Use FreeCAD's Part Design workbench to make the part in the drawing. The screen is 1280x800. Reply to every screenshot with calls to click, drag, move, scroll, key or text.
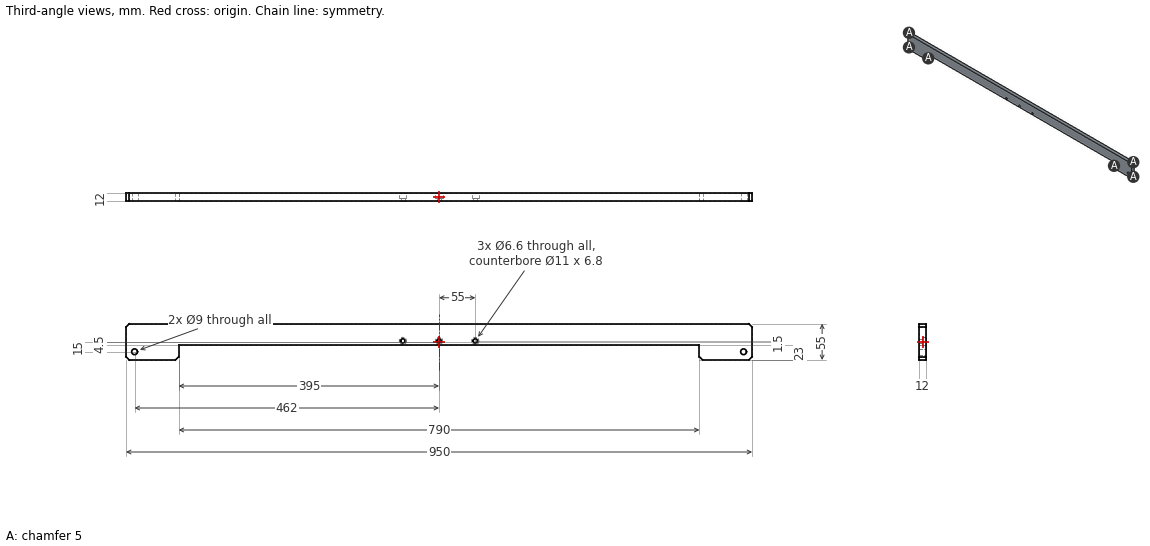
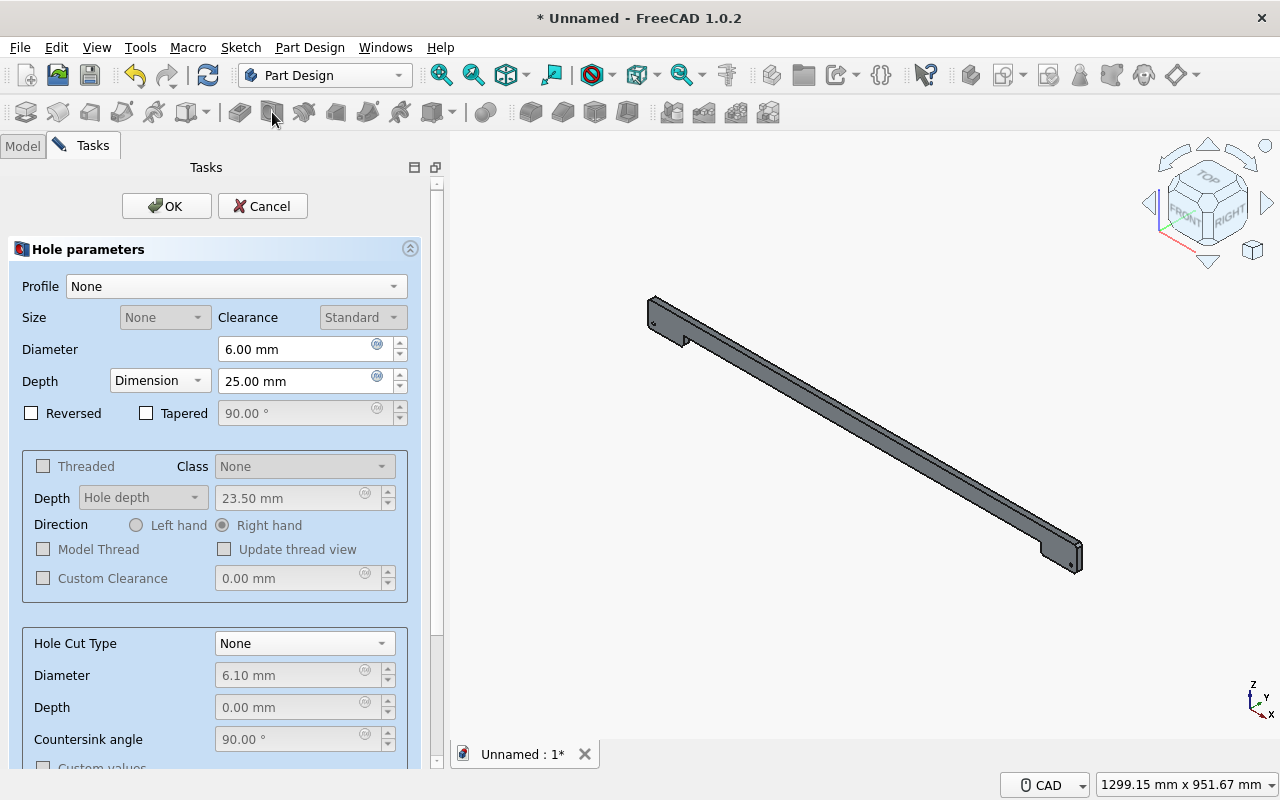
triple_click(305, 349)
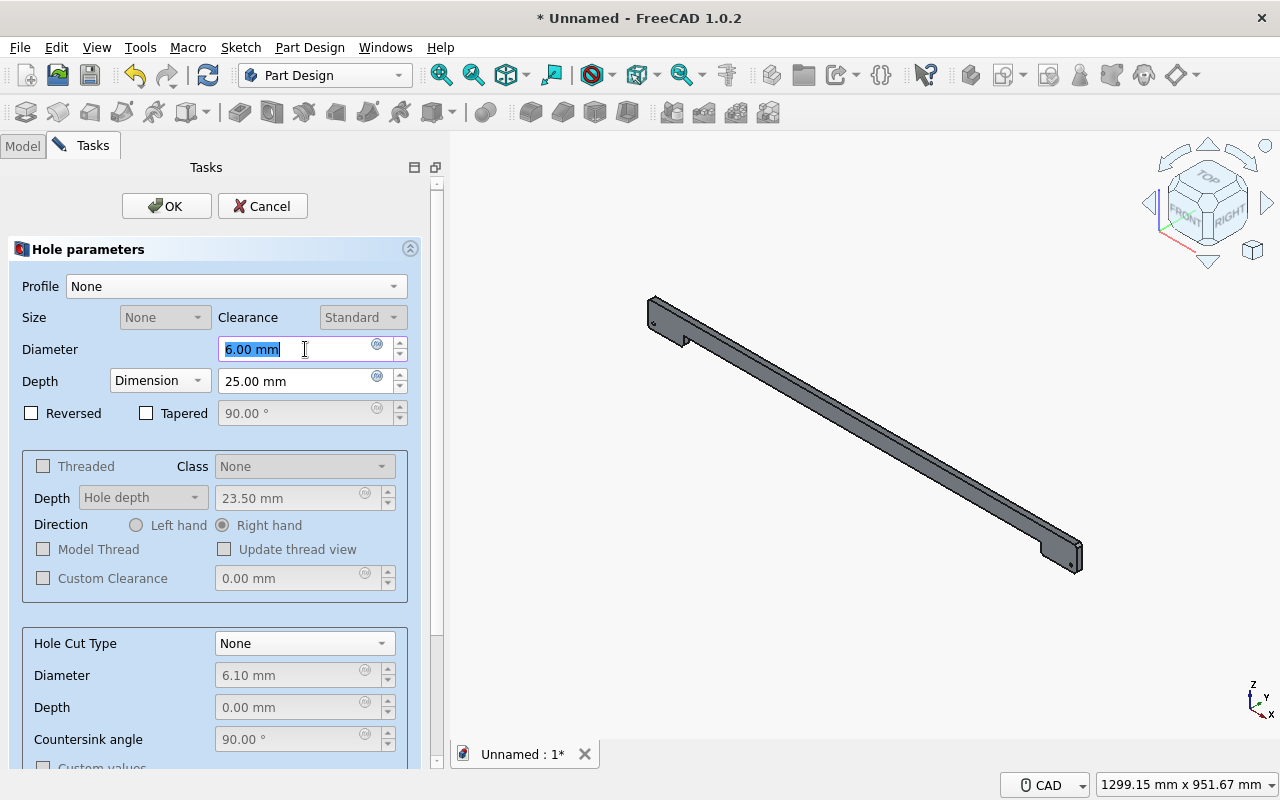
text(9)
key(Tab)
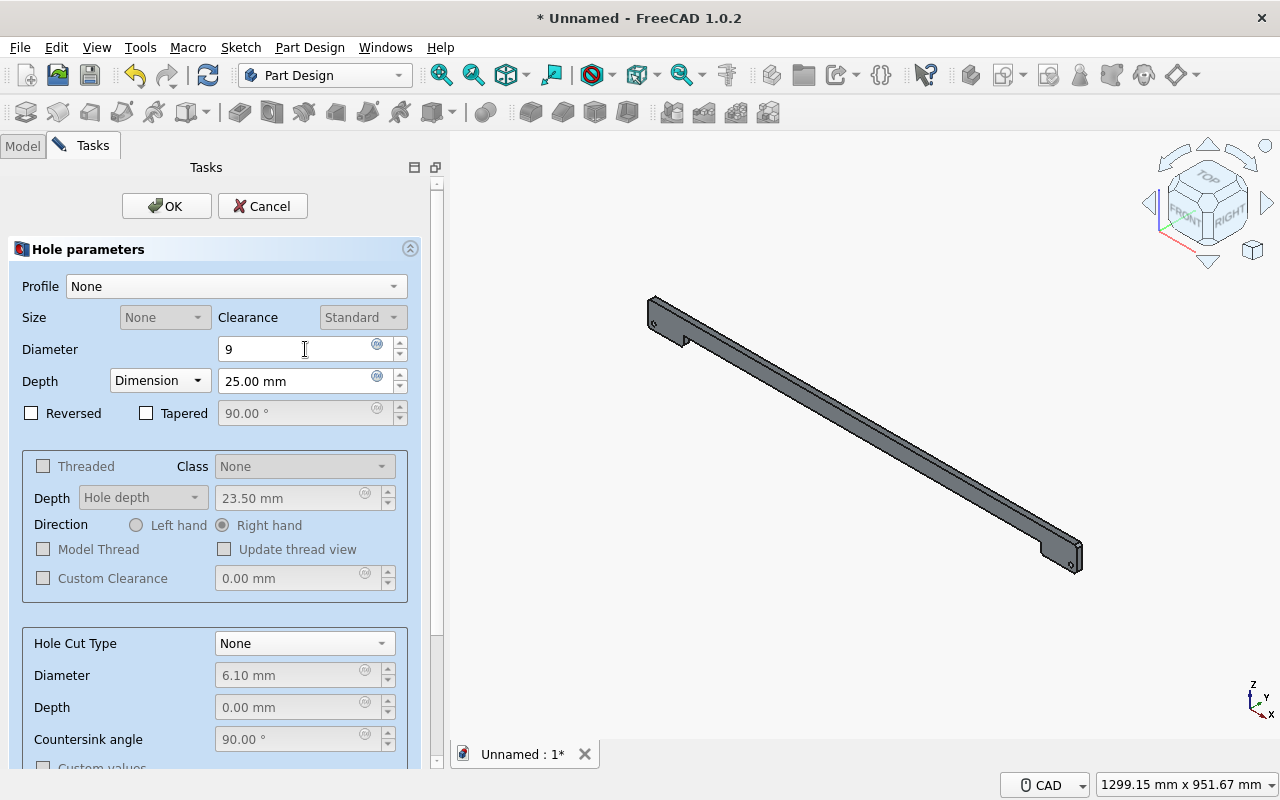
click(161, 380)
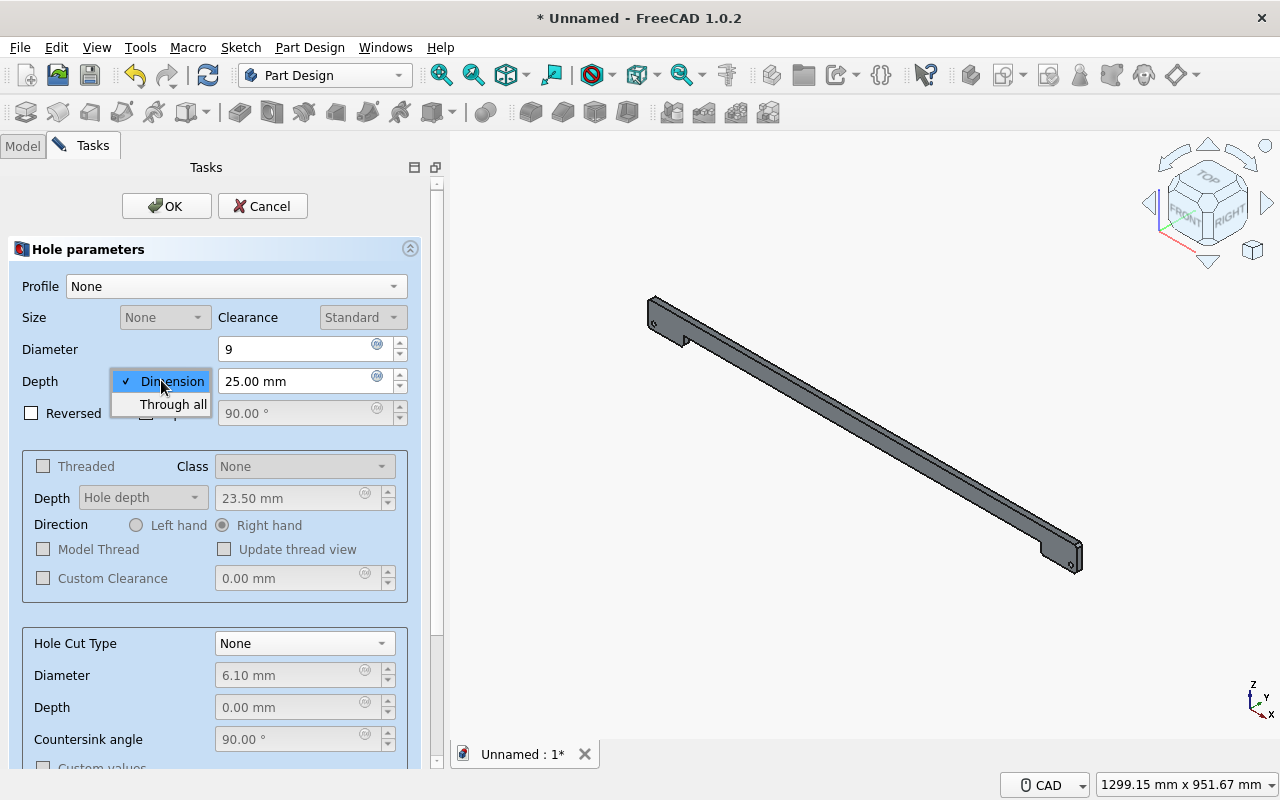
click(160, 404)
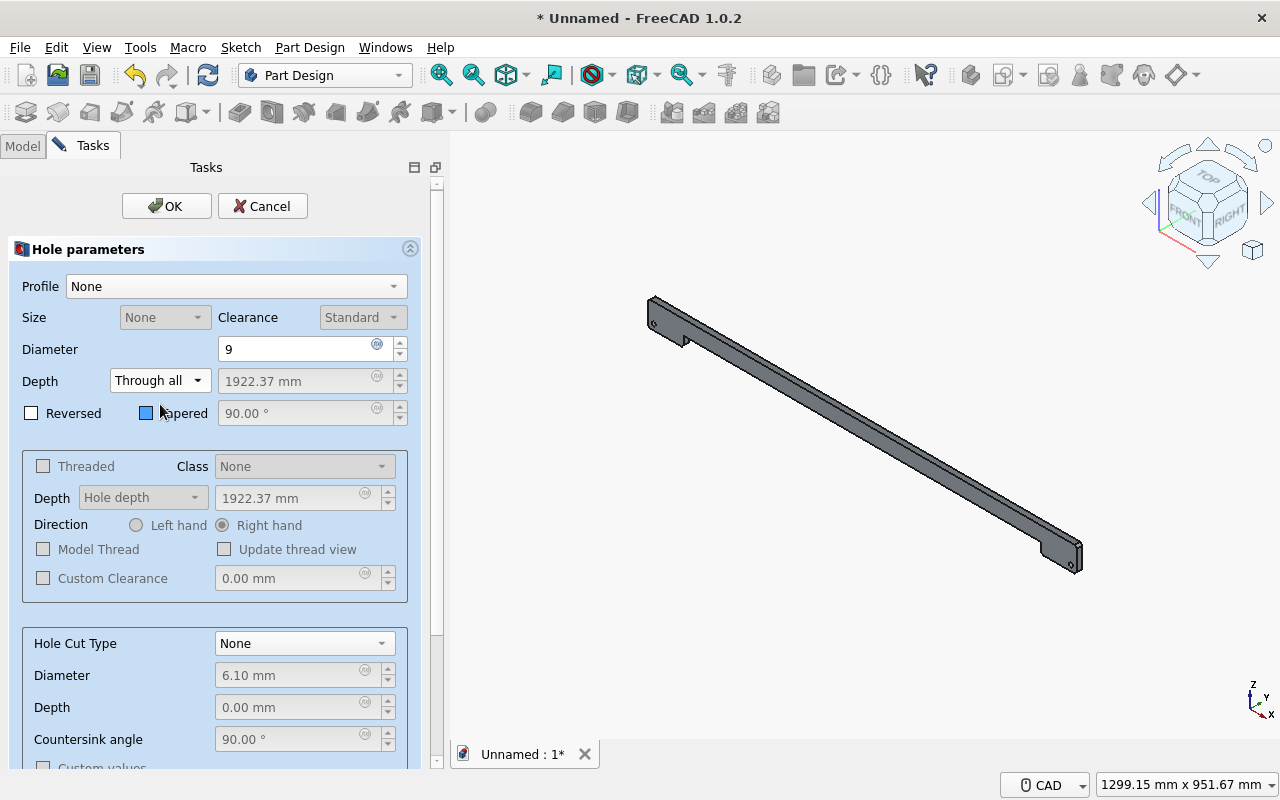
click(167, 206)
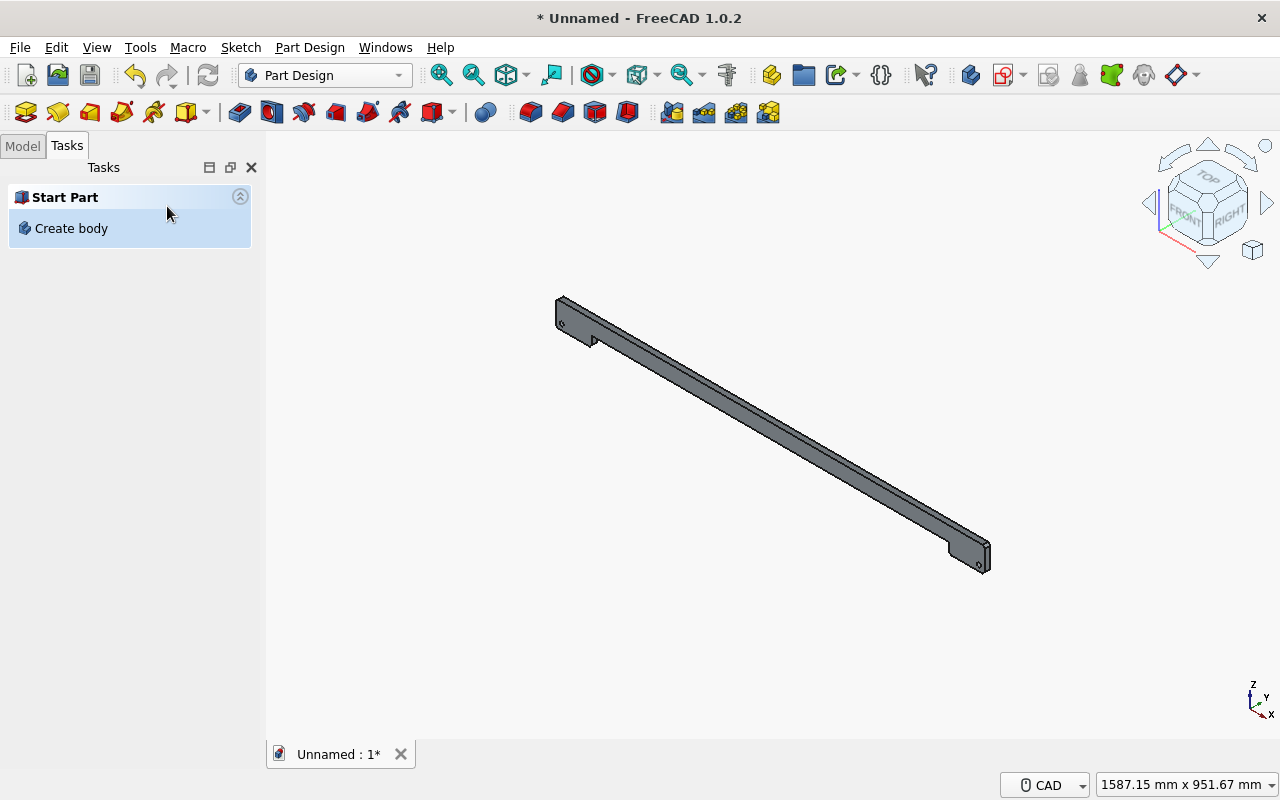
key(4)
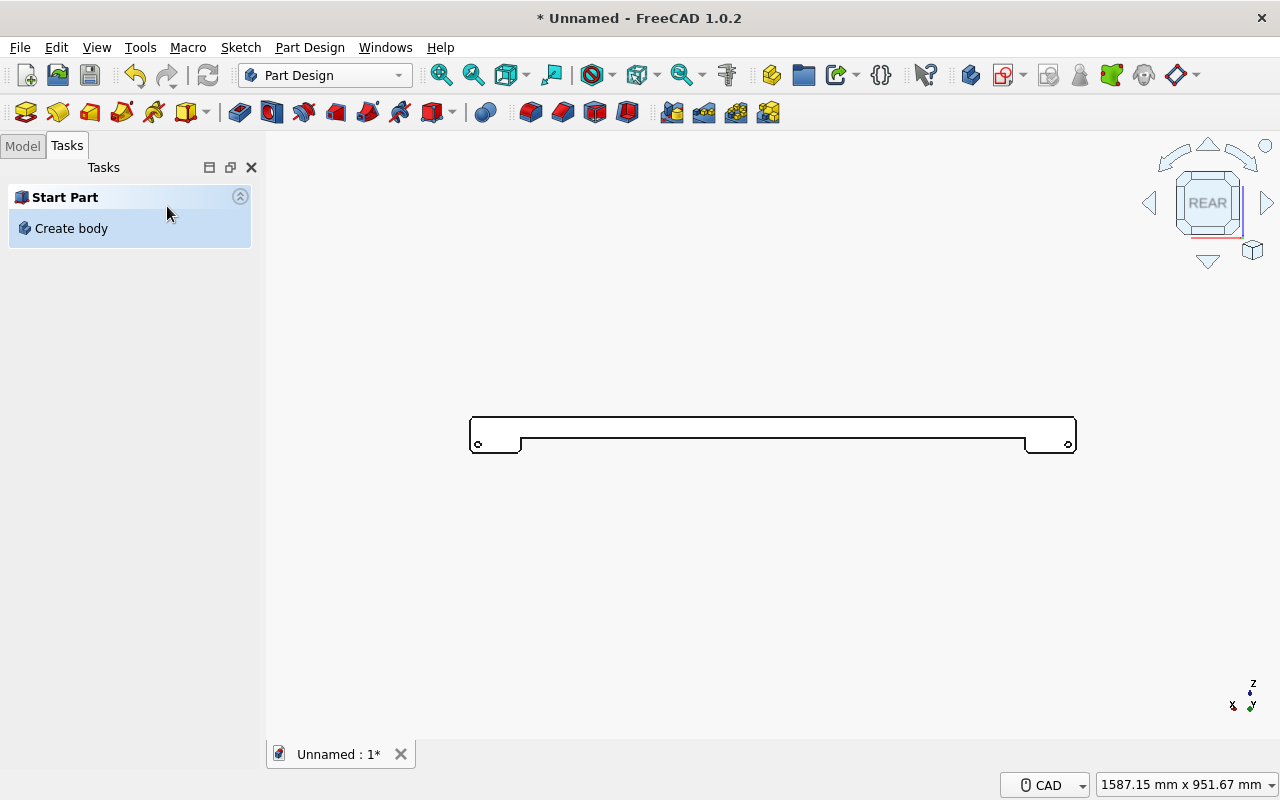
click(513, 429)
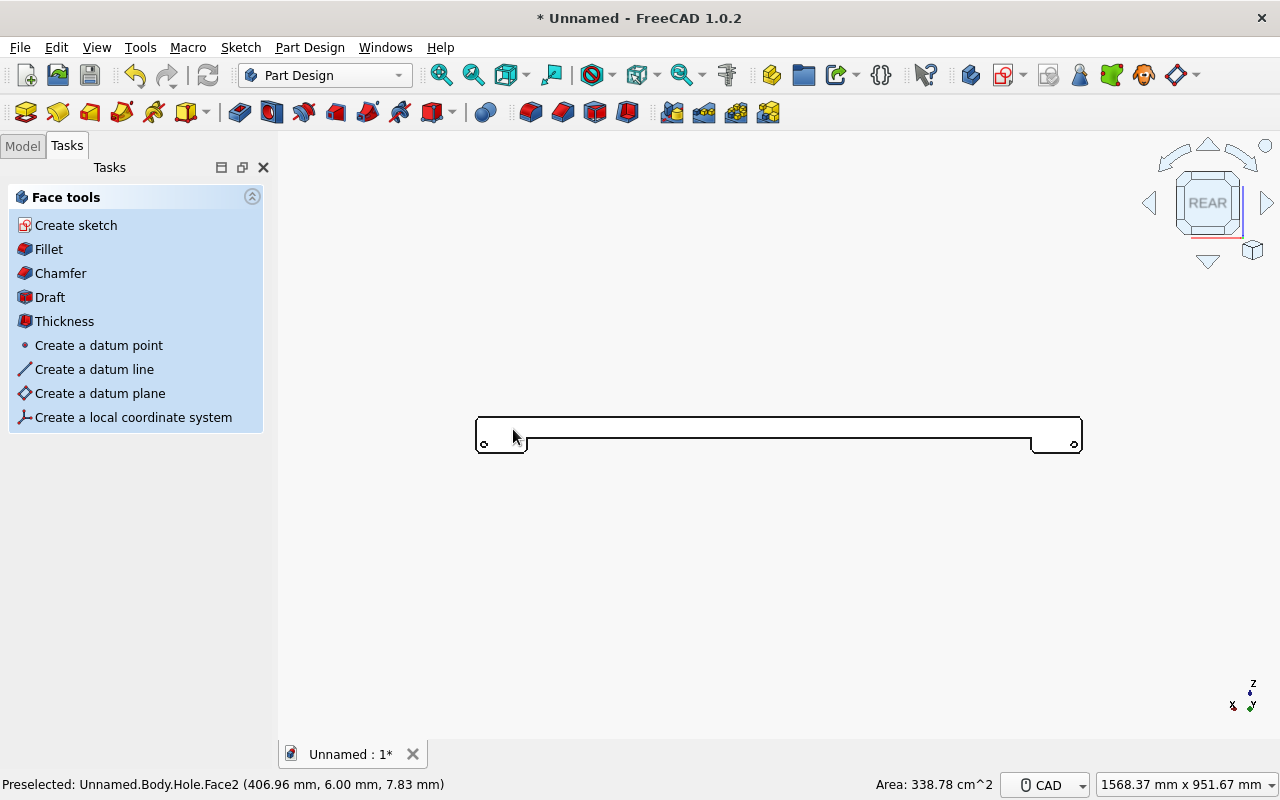
click(1004, 76)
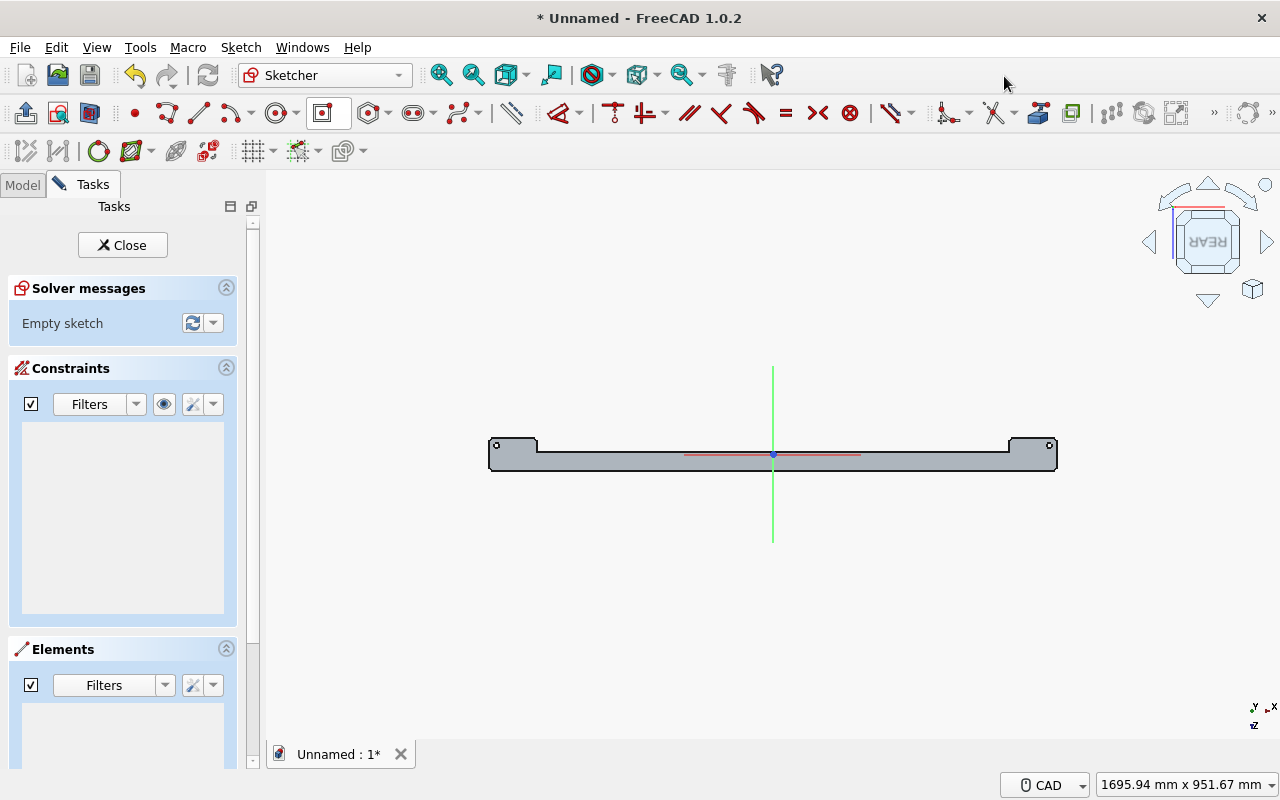
scroll(782, 456, up, 11)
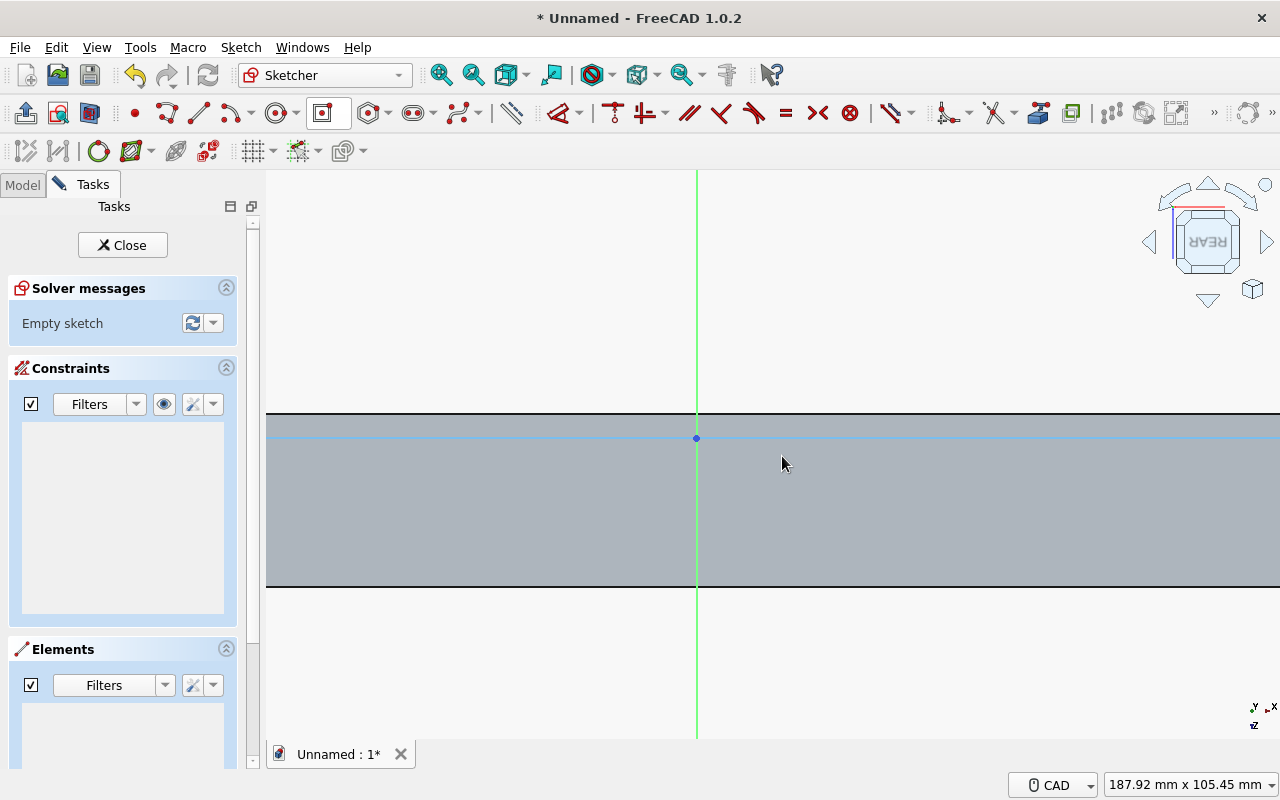
key(g)
key(c)